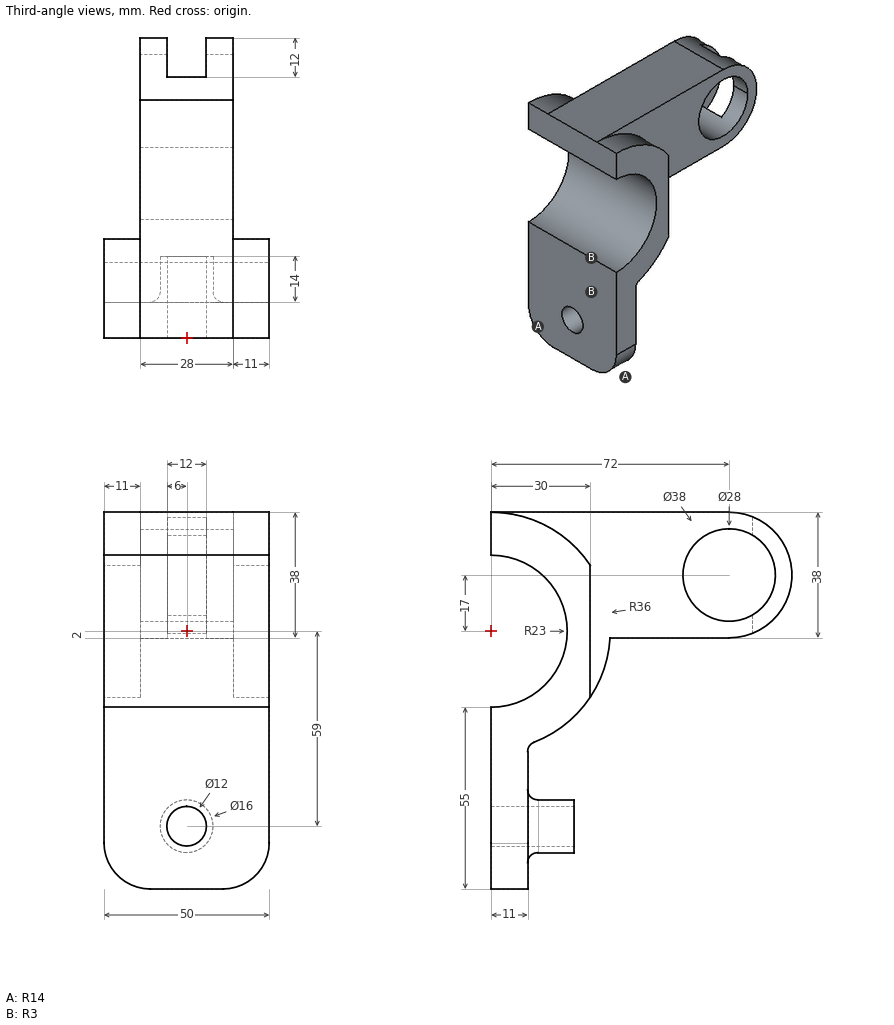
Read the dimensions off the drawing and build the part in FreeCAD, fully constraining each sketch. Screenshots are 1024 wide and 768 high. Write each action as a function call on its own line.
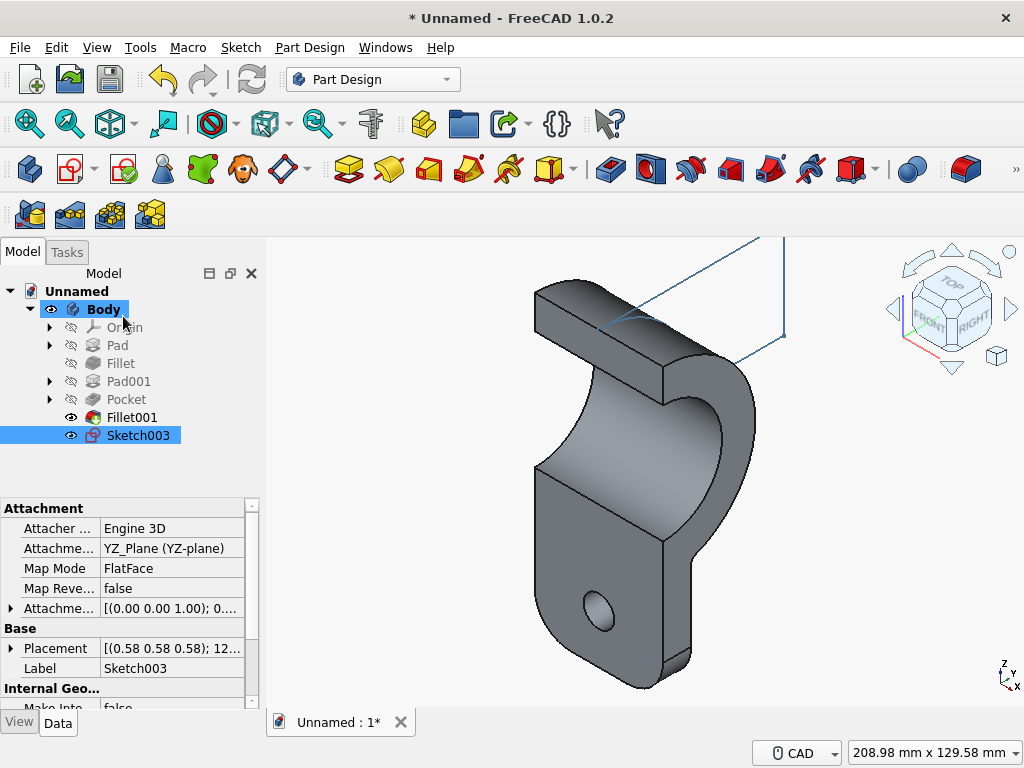
click(350, 170)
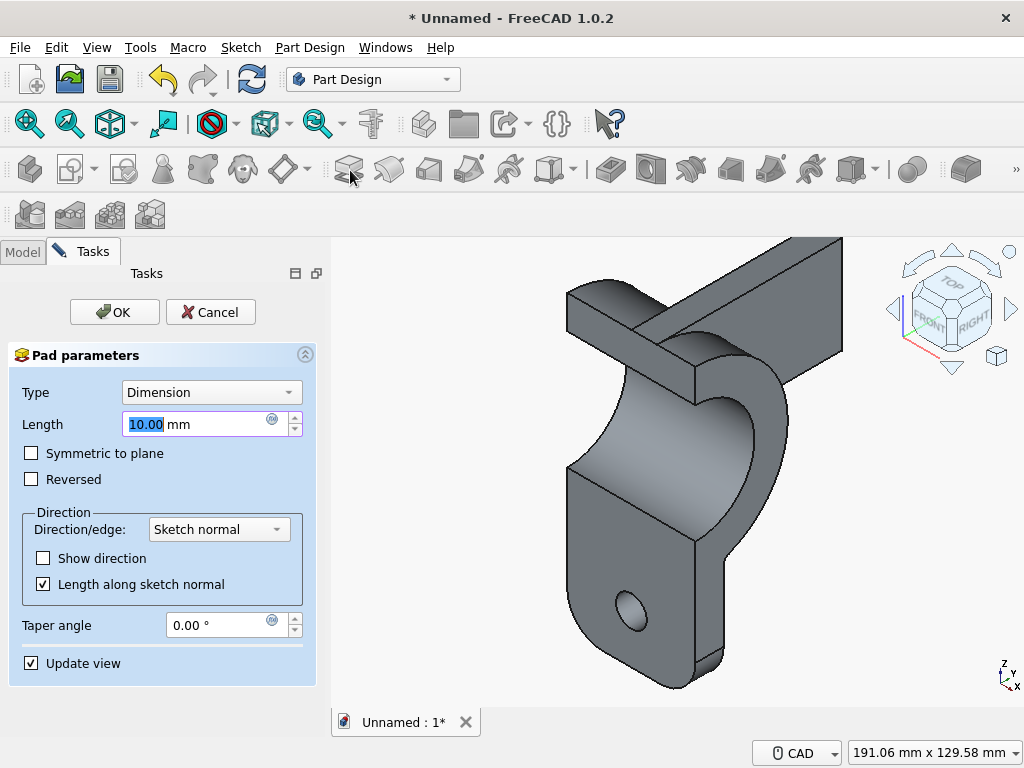
text(28)
key(Tab)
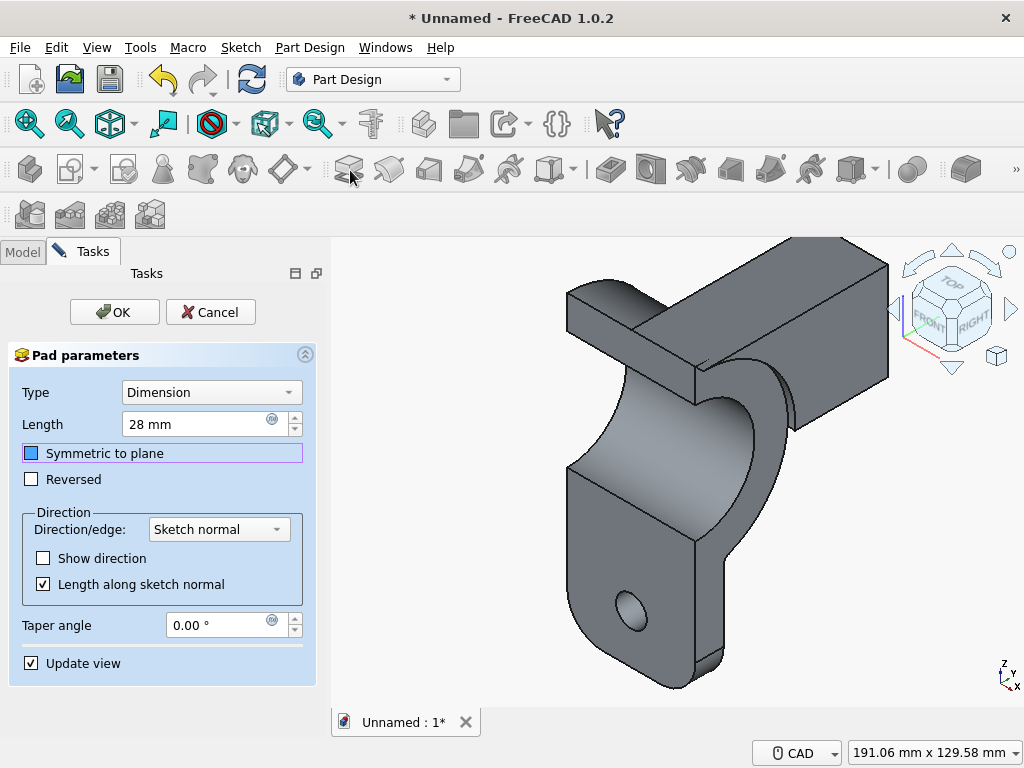
click(30, 453)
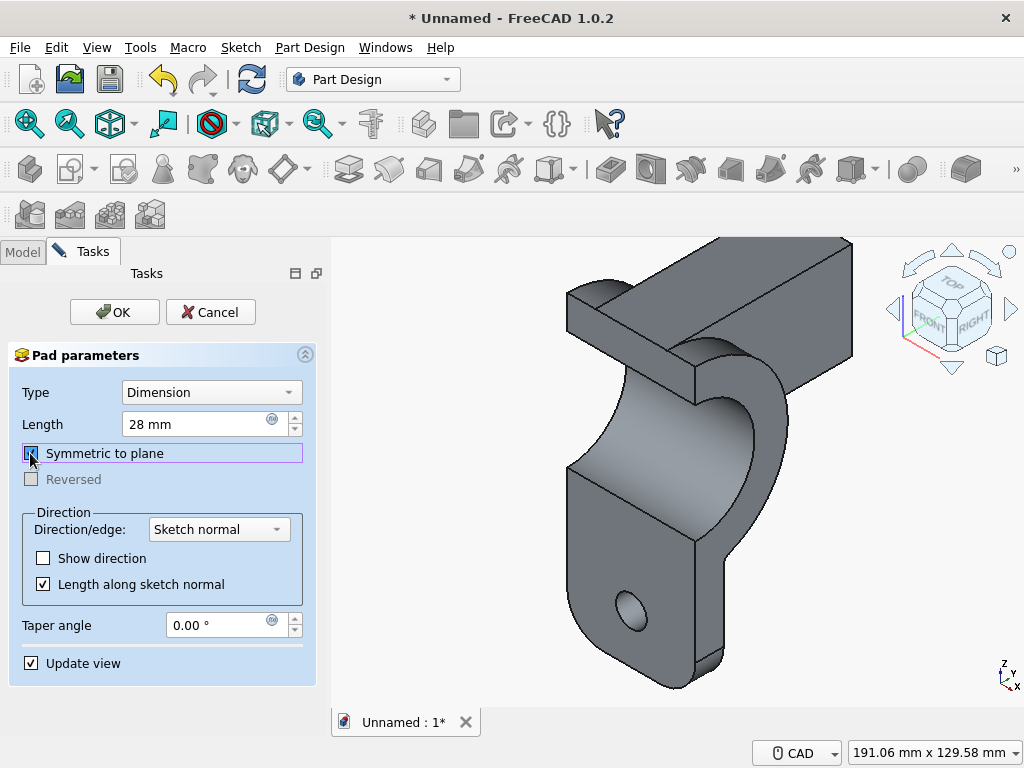
click(115, 312)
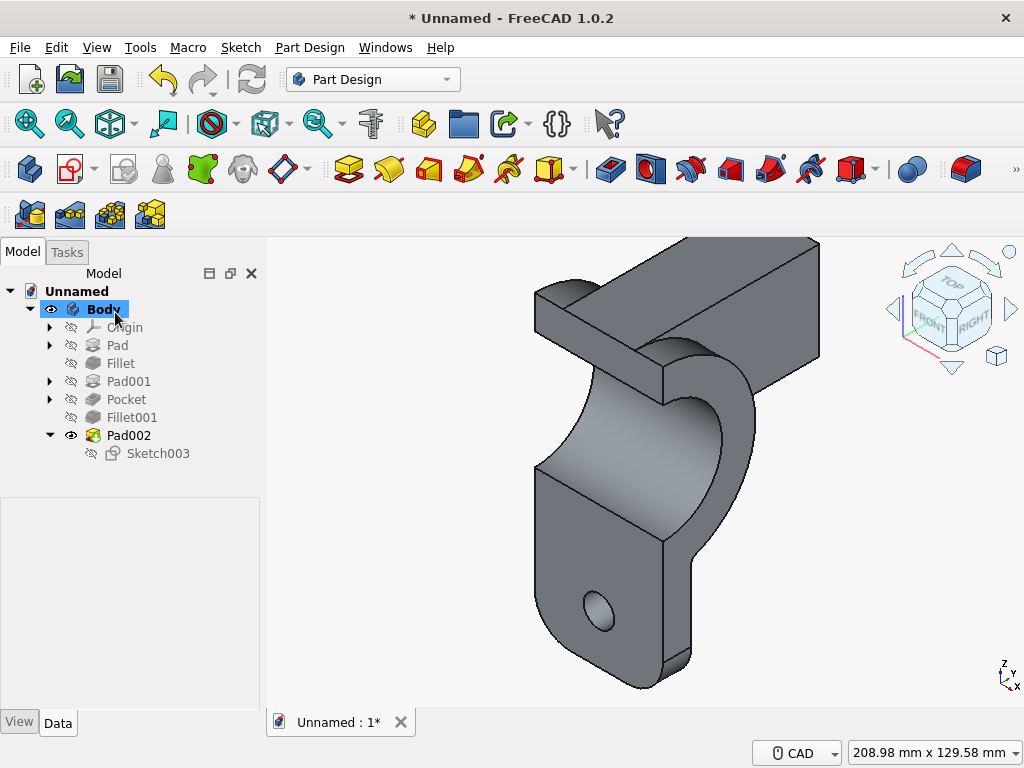
click(30, 124)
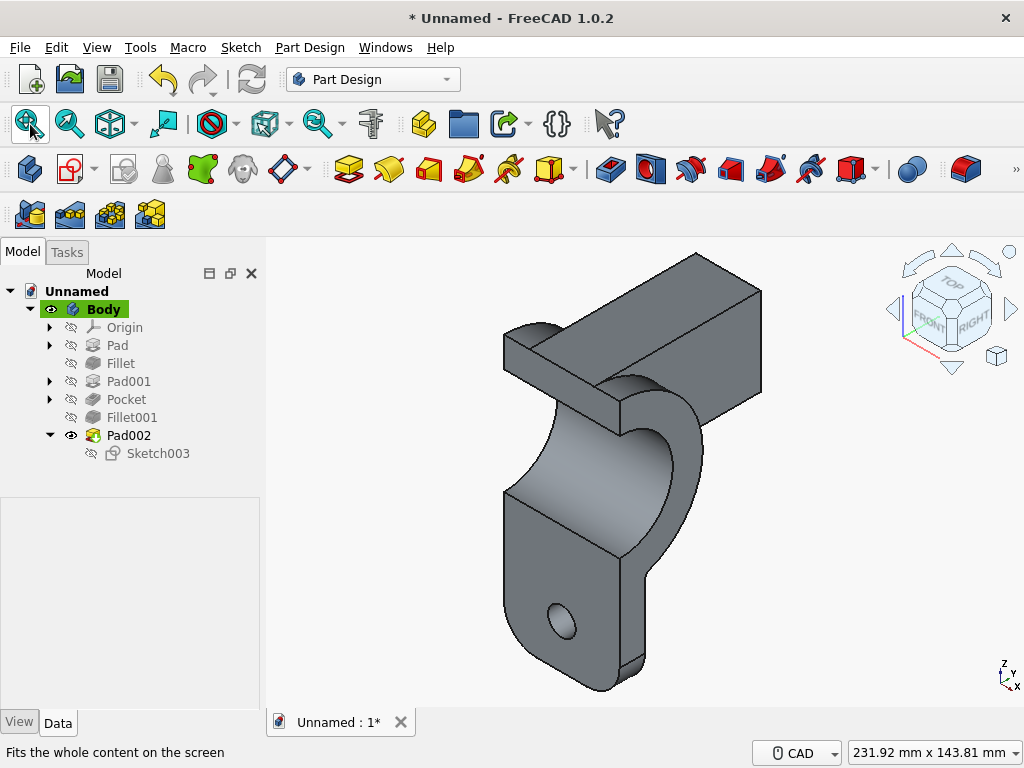
click(70, 170)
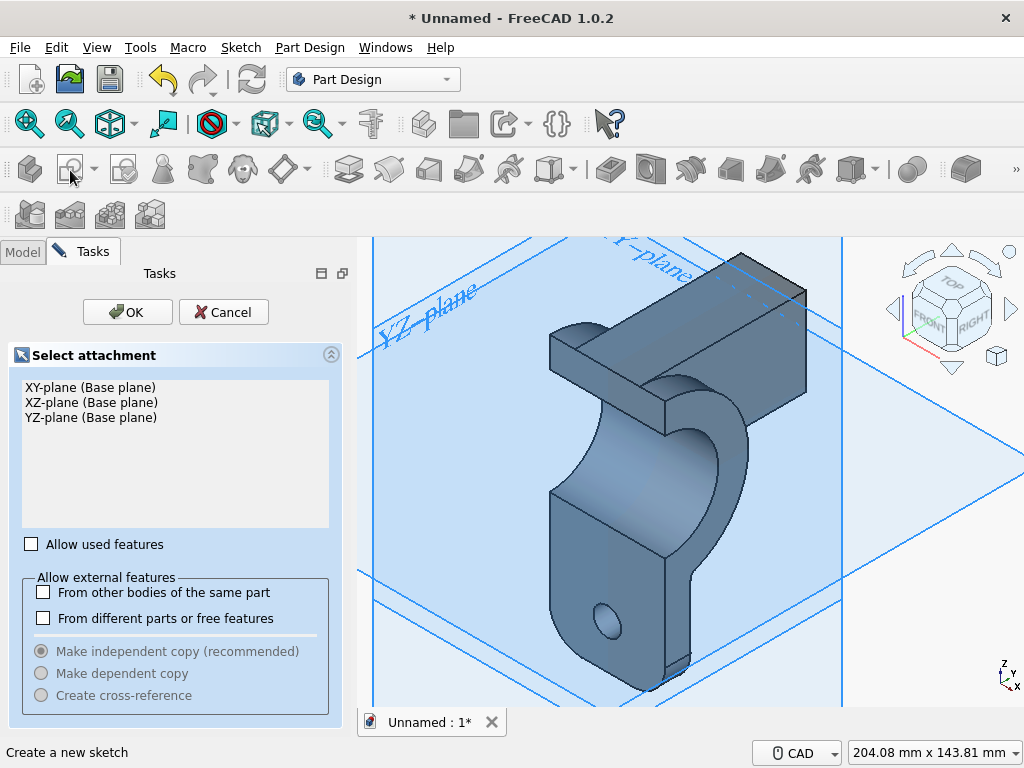
click(82, 418)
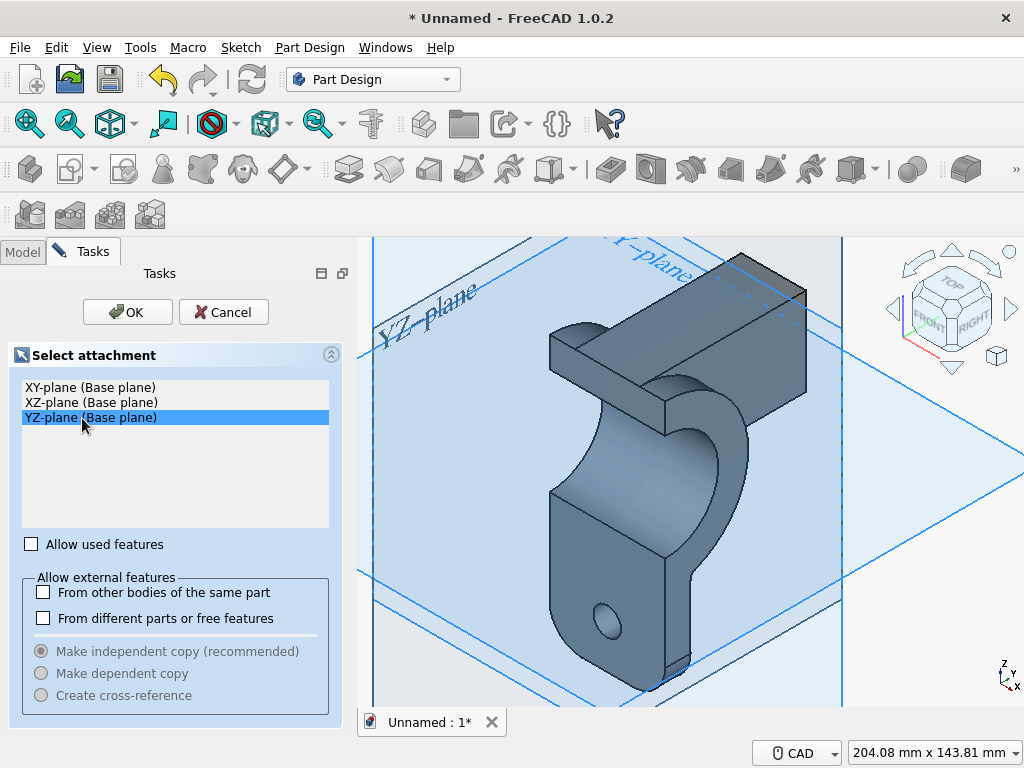
click(128, 312)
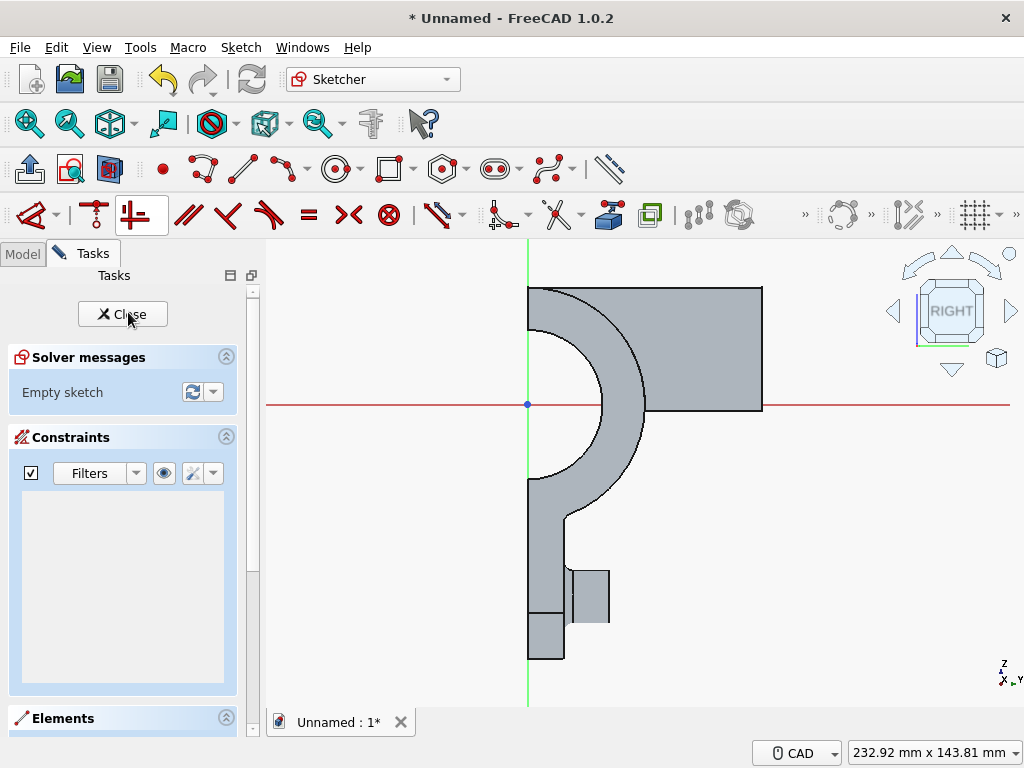
click(110, 170)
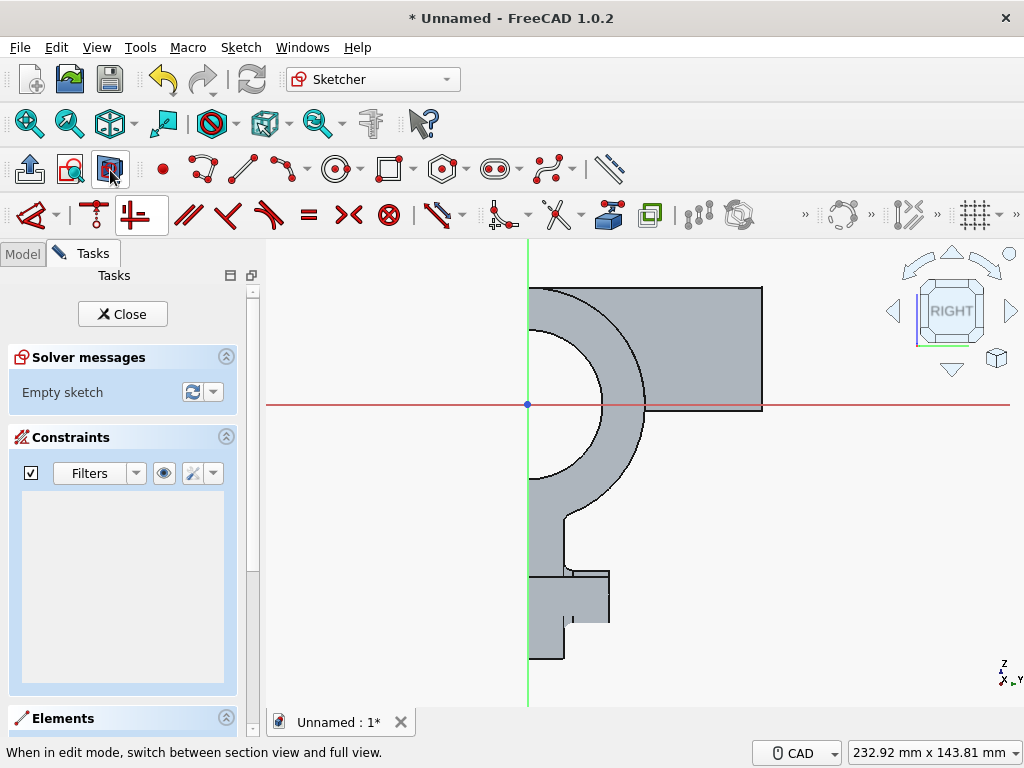
scroll(859, 267, up, 1)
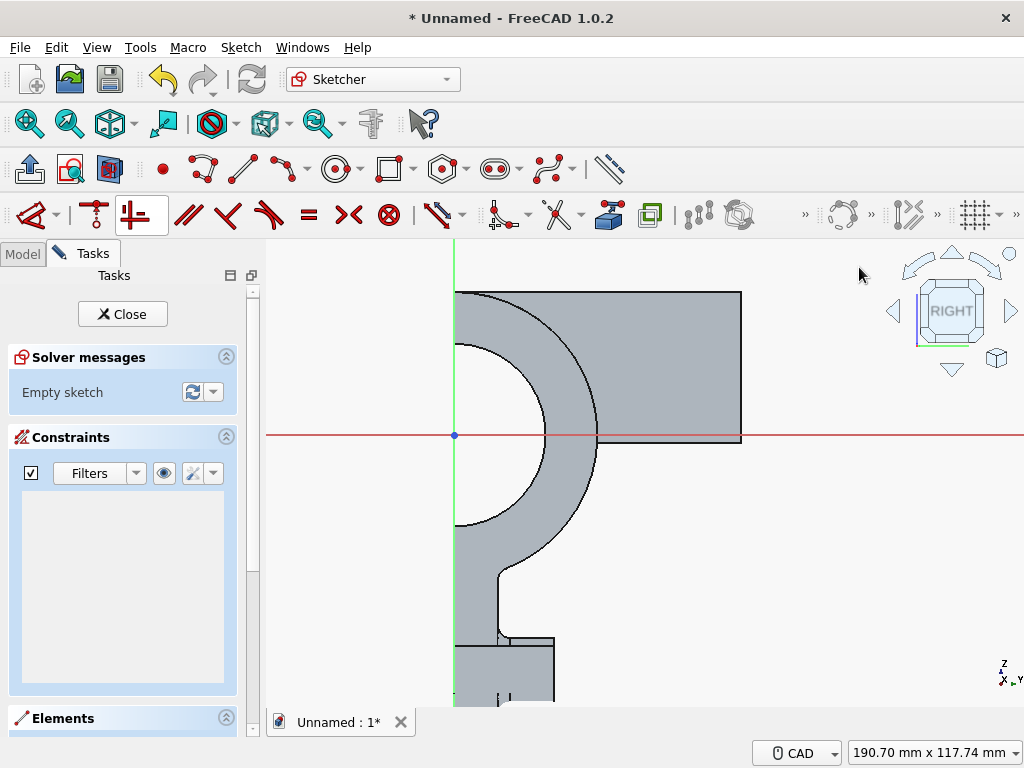
click(336, 170)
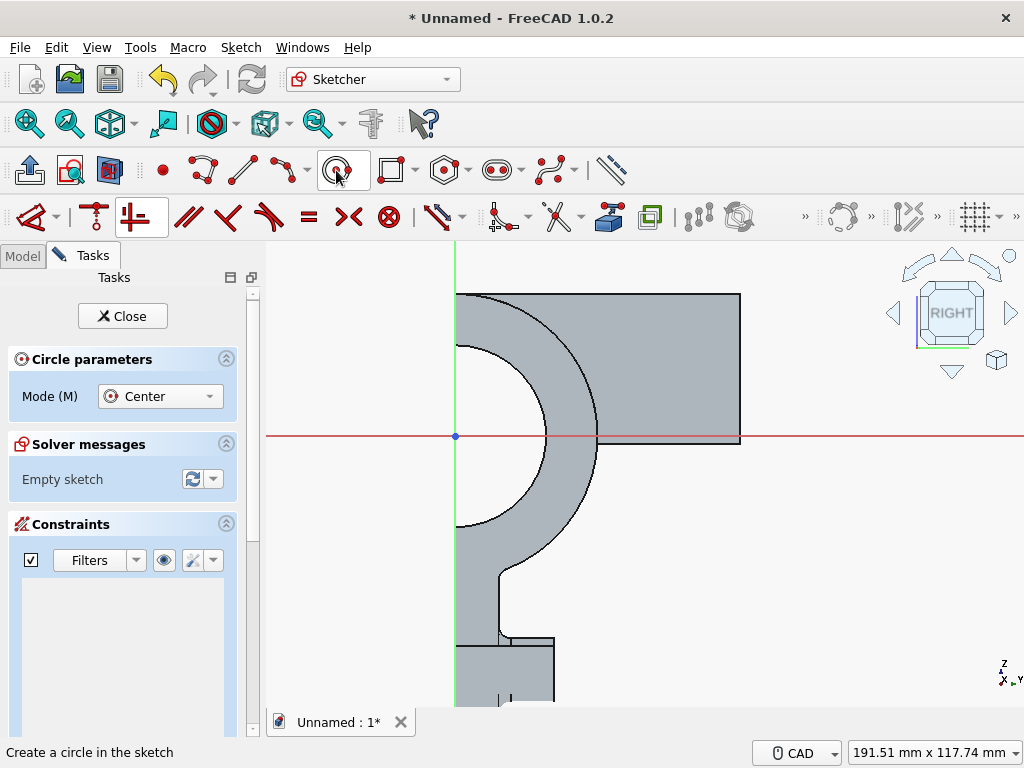
click(740, 369)
move(793, 316)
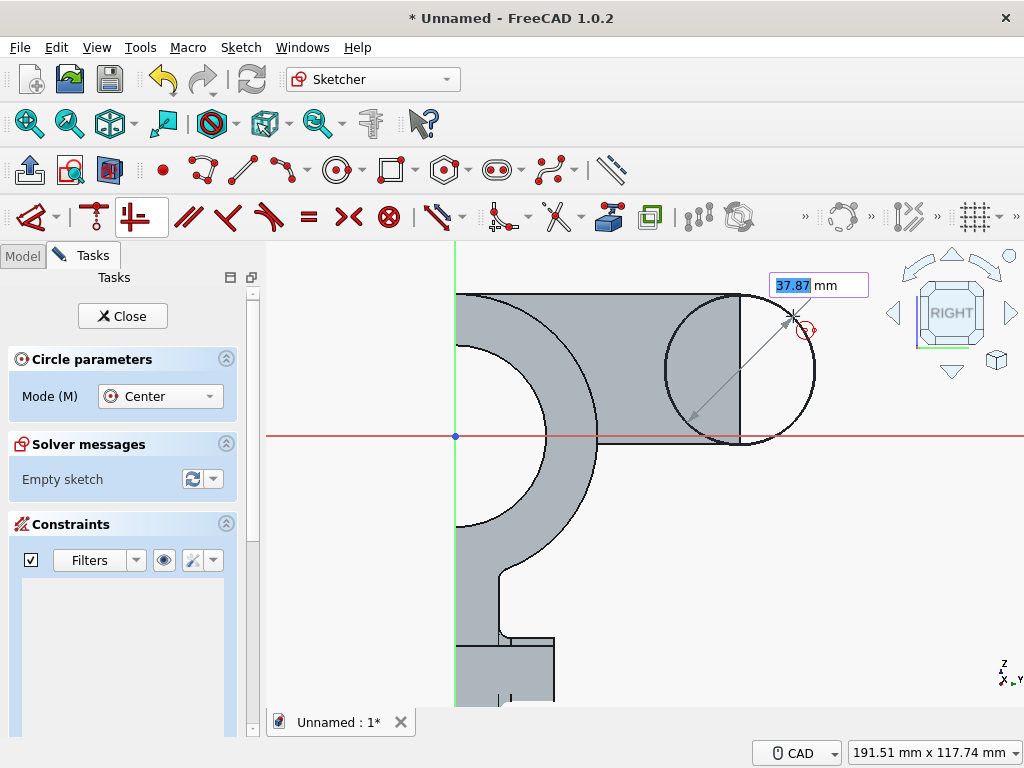
text(38)
key(Return)
key(Escape)